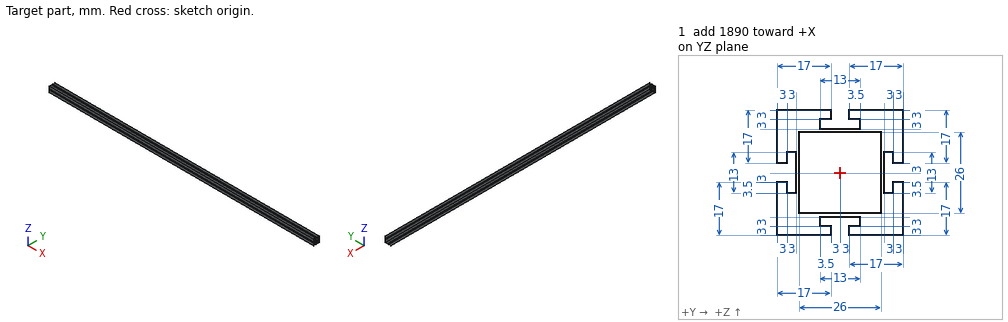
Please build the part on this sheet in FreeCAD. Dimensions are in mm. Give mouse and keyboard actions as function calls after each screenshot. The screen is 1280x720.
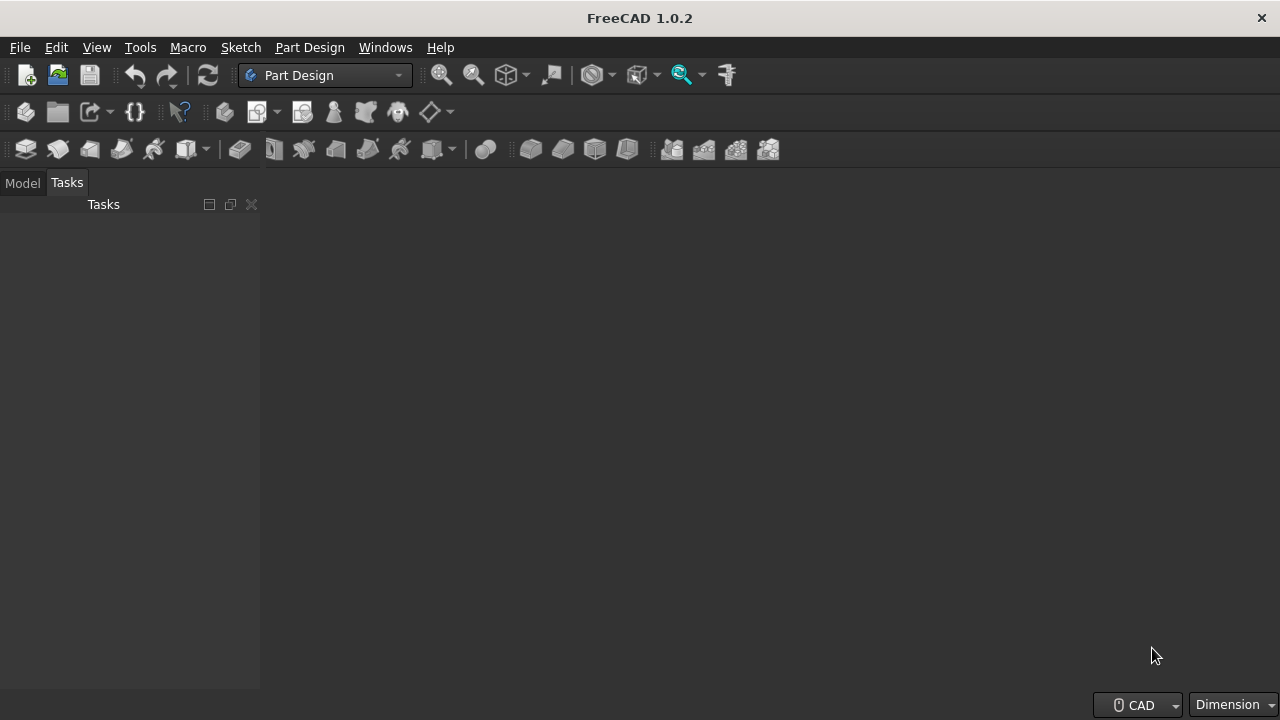
click(546, 112)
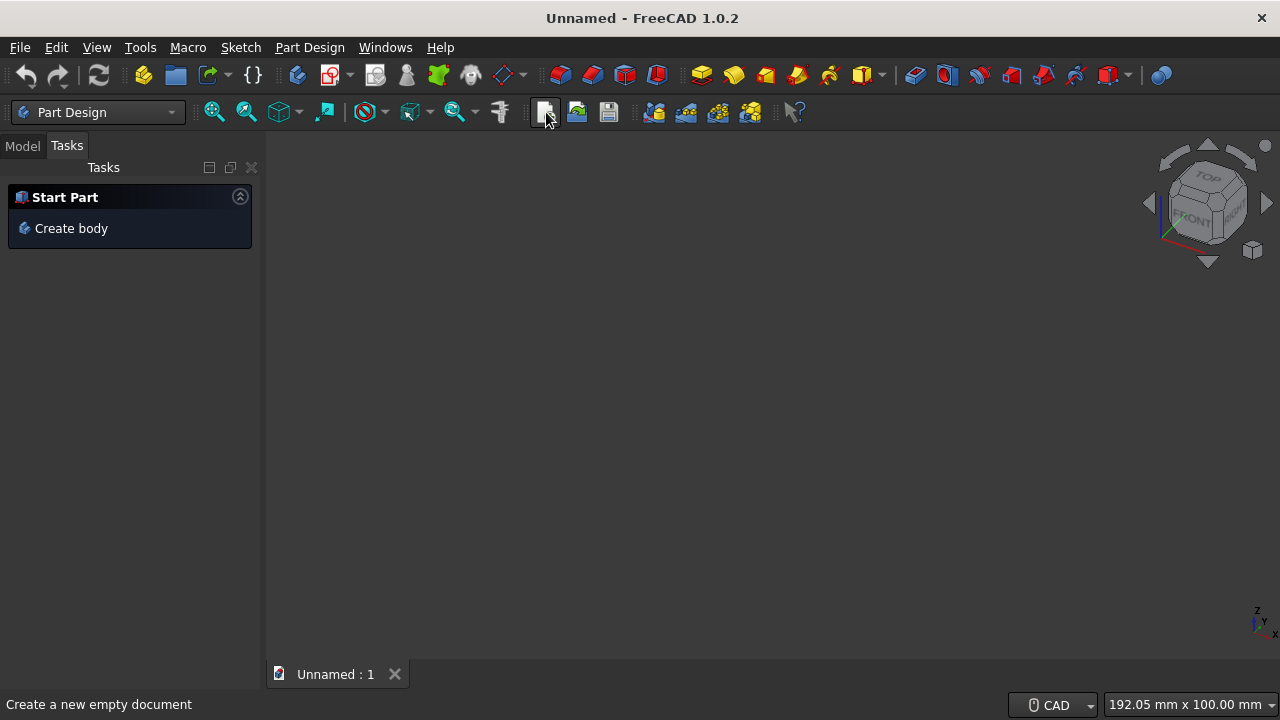
click(330, 76)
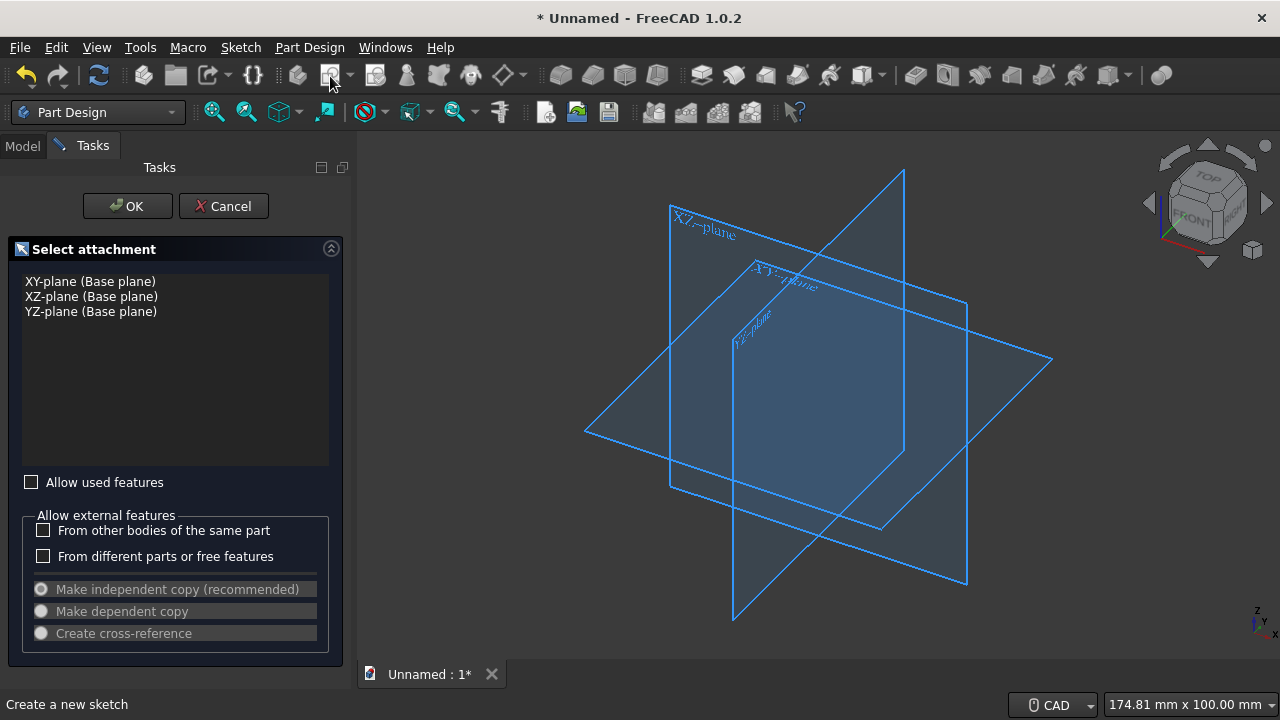
click(82, 312)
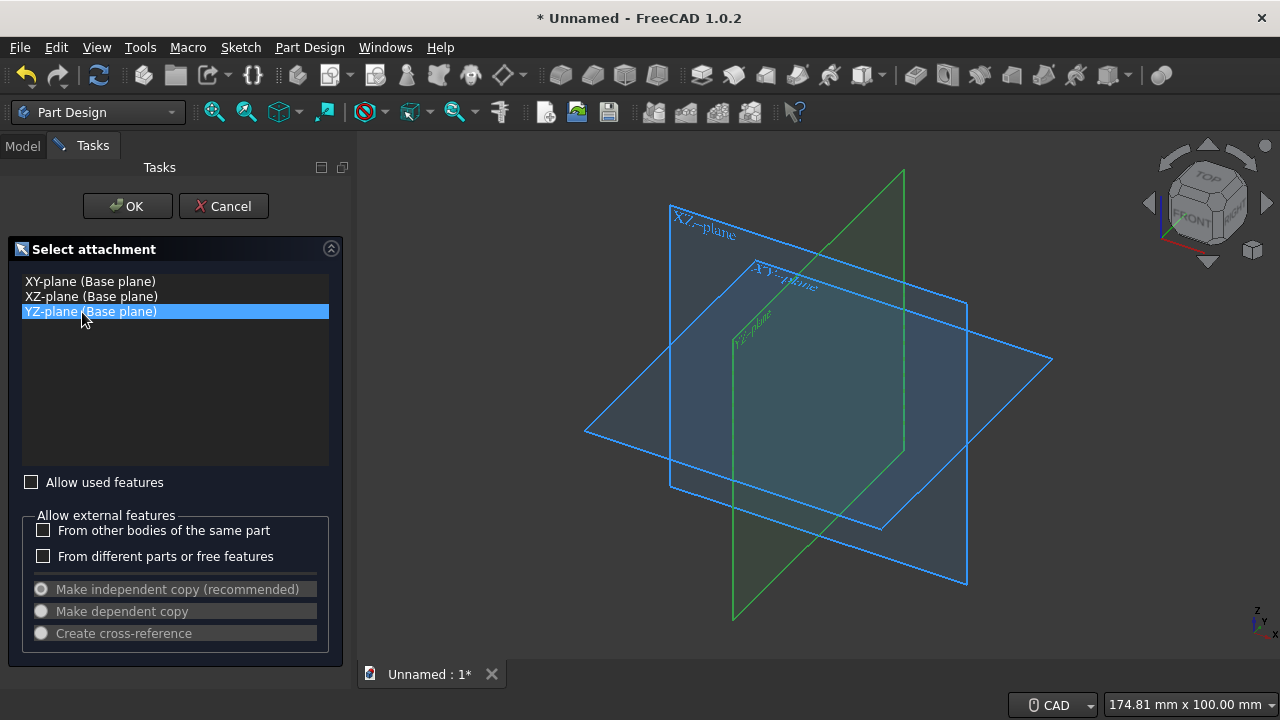
click(128, 206)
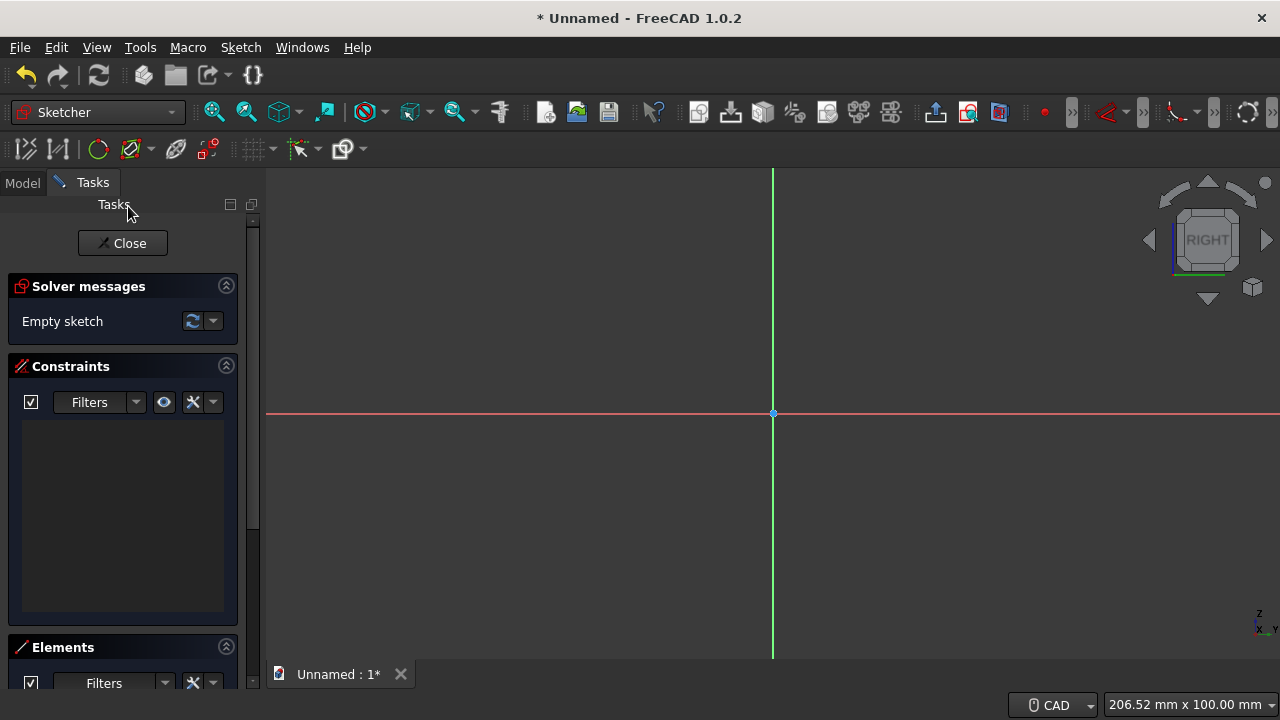
scroll(912, 413, up, 2)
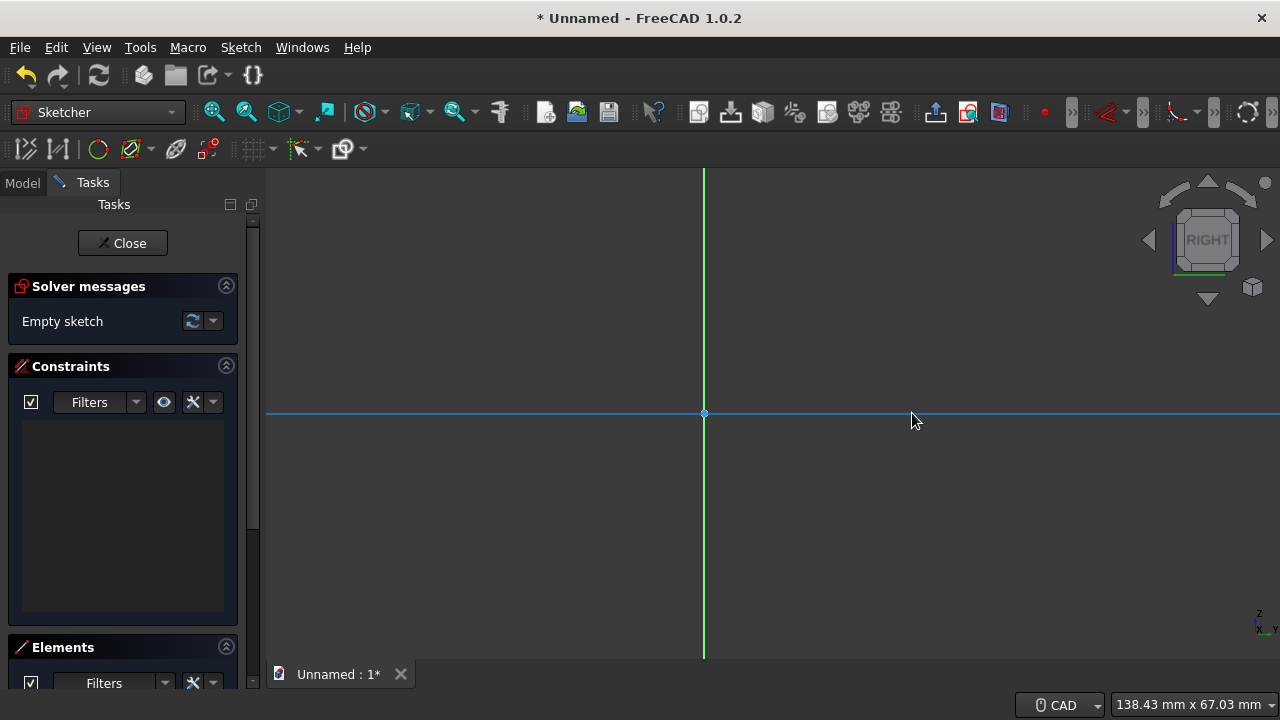
key(g)
key(m)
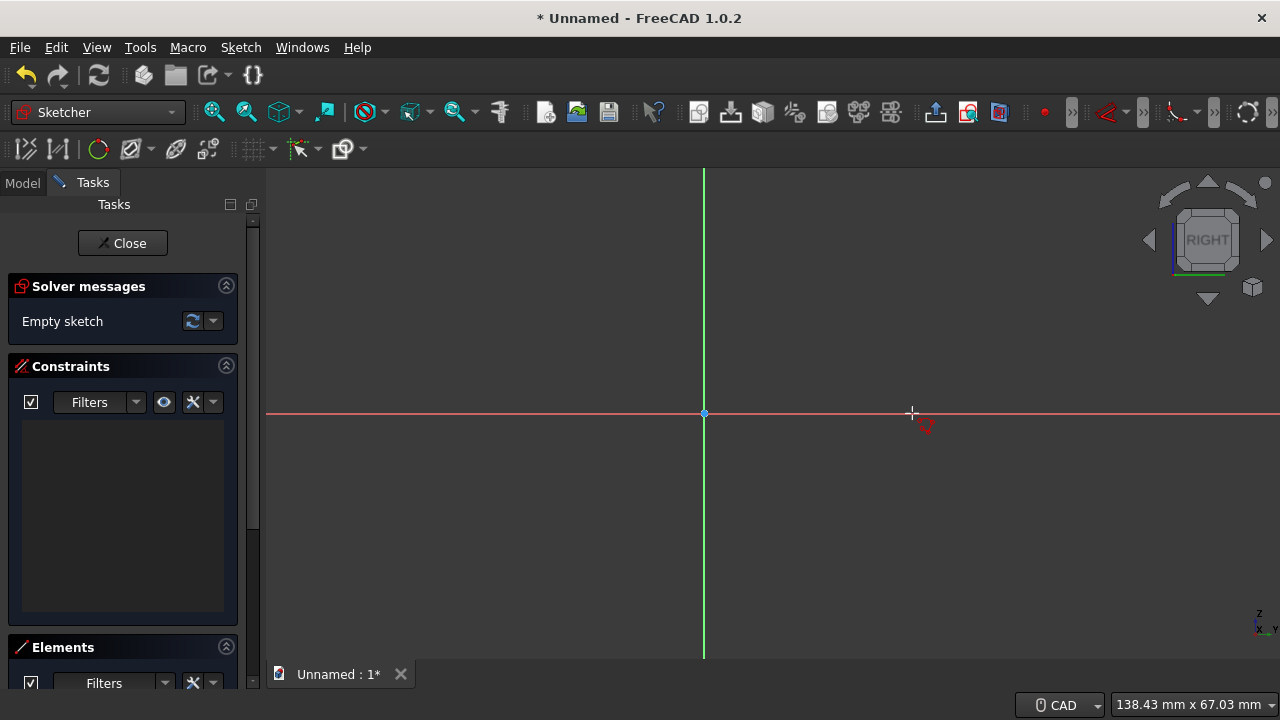
click(602, 366)
click(602, 461)
click(580, 461)
click(580, 435)
click(558, 435)
click(558, 560)
click(682, 560)
click(682, 538)
click(657, 538)
click(657, 516)
click(752, 516)
click(752, 538)
click(726, 538)
click(726, 560)
click(851, 560)
click(851, 435)
click(829, 435)
click(829, 461)
click(807, 461)
click(807, 366)
click(829, 366)
click(829, 392)
click(851, 392)
click(851, 267)
click(726, 267)
click(726, 289)
click(752, 289)
click(752, 311)
click(657, 311)
click(657, 289)
click(682, 289)
click(682, 267)
click(558, 267)
click(558, 392)
click(580, 392)
click(580, 366)
click(602, 367)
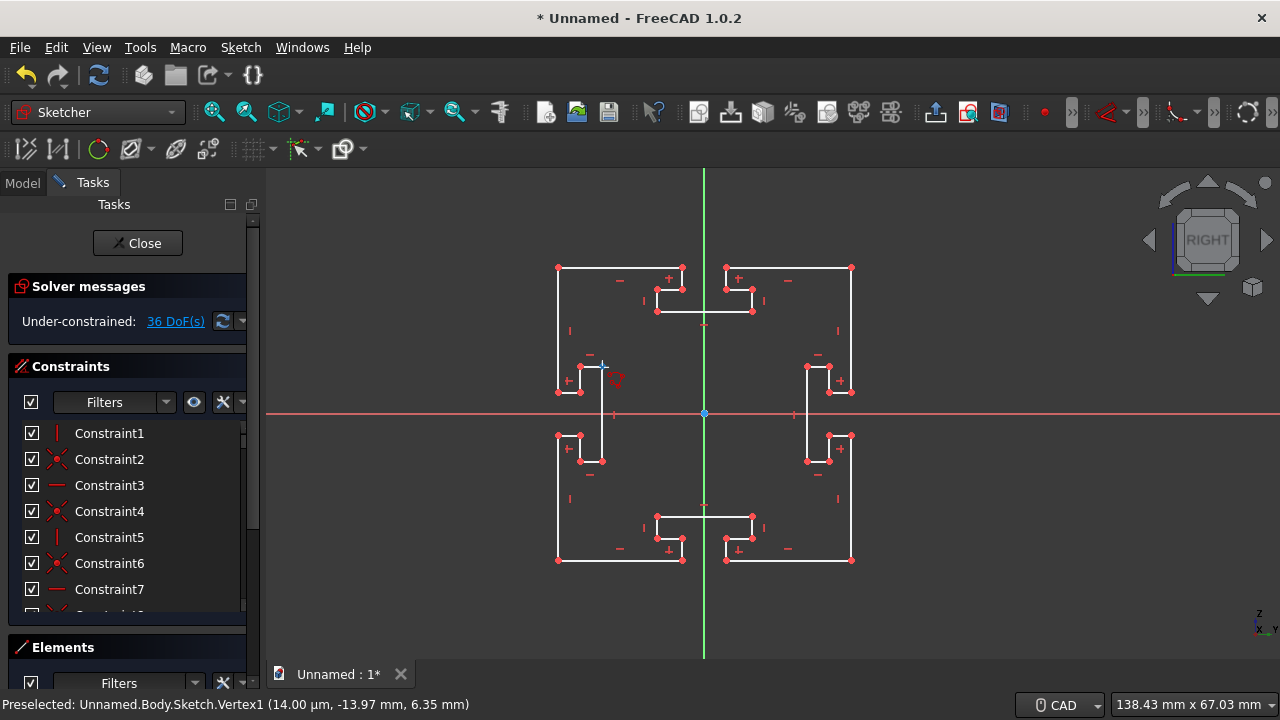
key(g)
key(v)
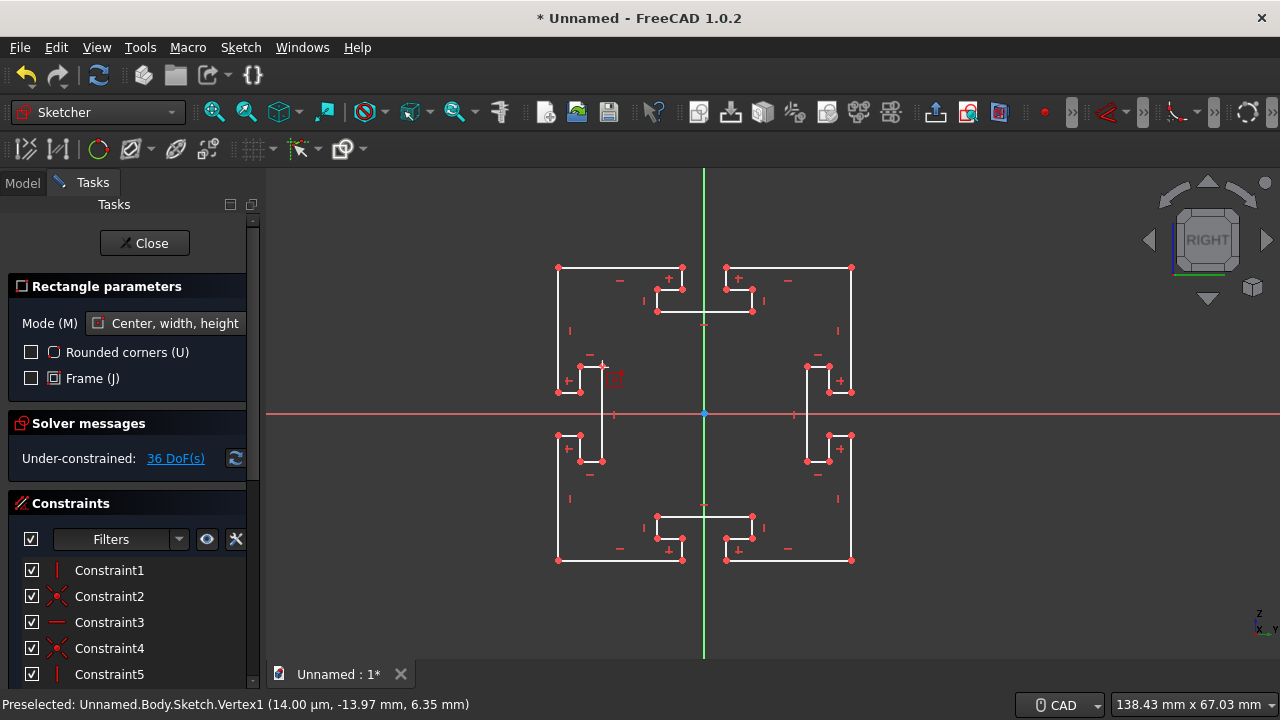
click(704, 414)
click(800, 318)
key(Escape)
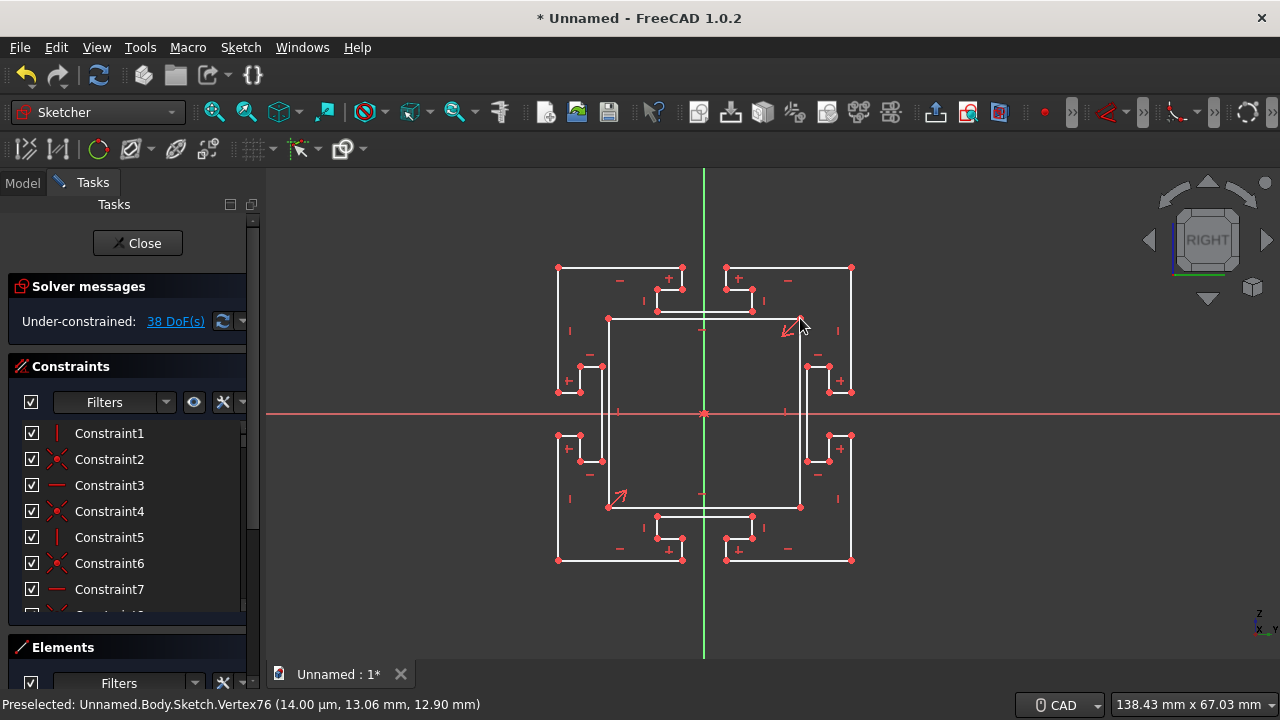
scroll(591, 462, up, 3)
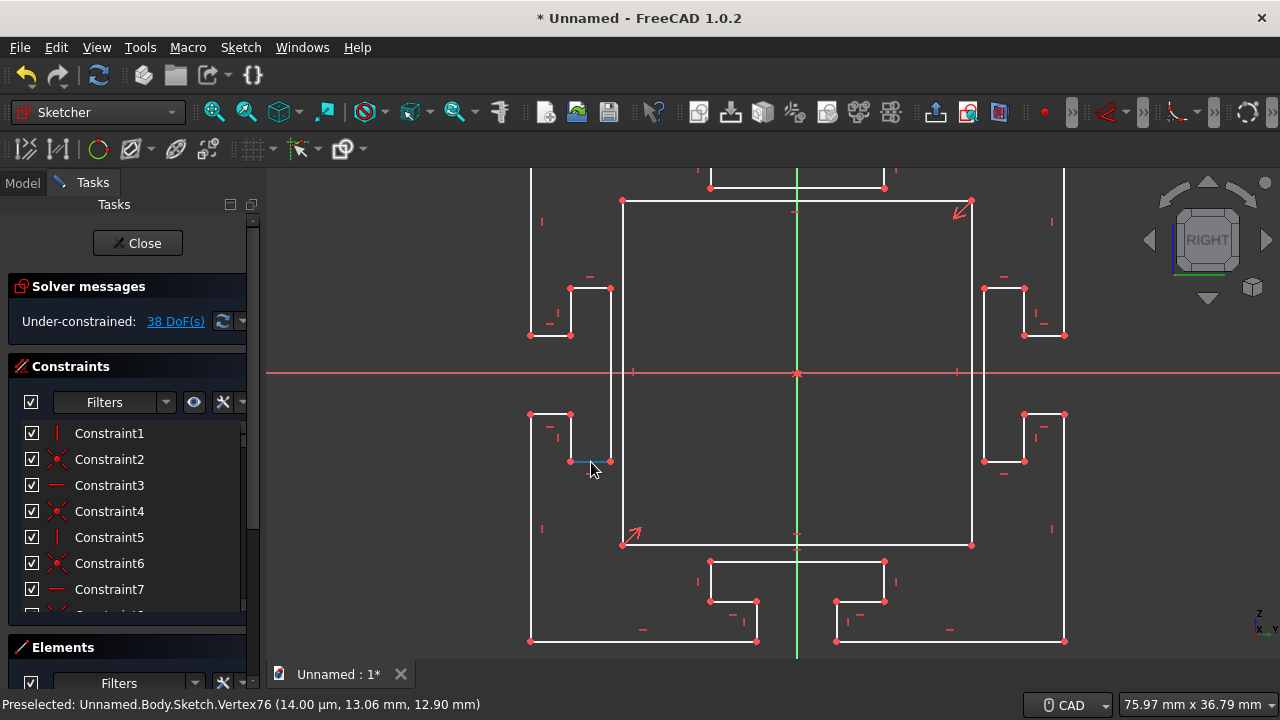
click(591, 462)